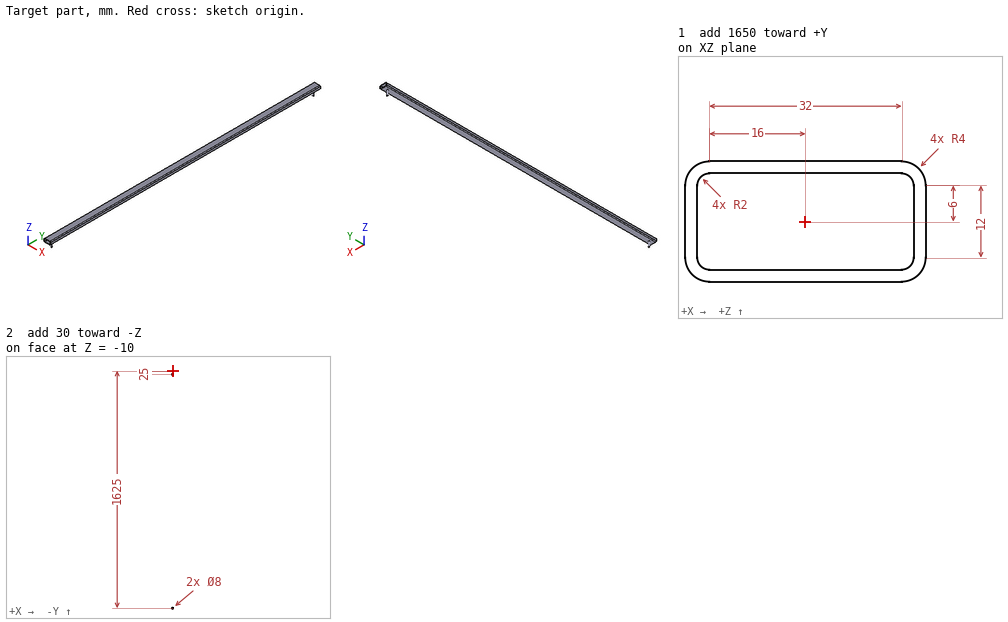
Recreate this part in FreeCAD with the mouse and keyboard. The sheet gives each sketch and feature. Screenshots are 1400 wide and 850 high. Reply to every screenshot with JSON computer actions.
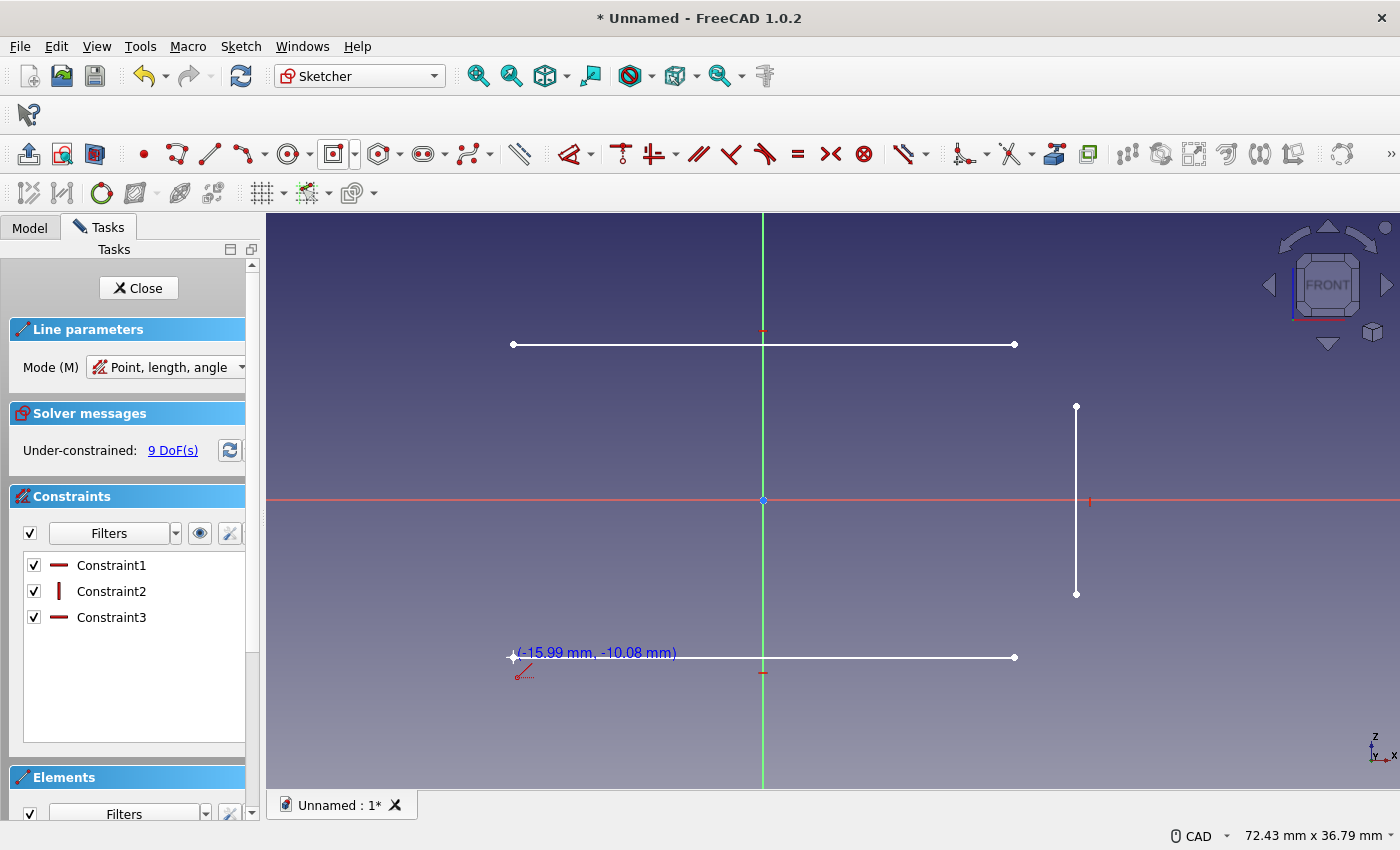
{"action": "left_click", "coordinate": [450, 594]}
{"action": "left_click", "coordinate": [450, 406]}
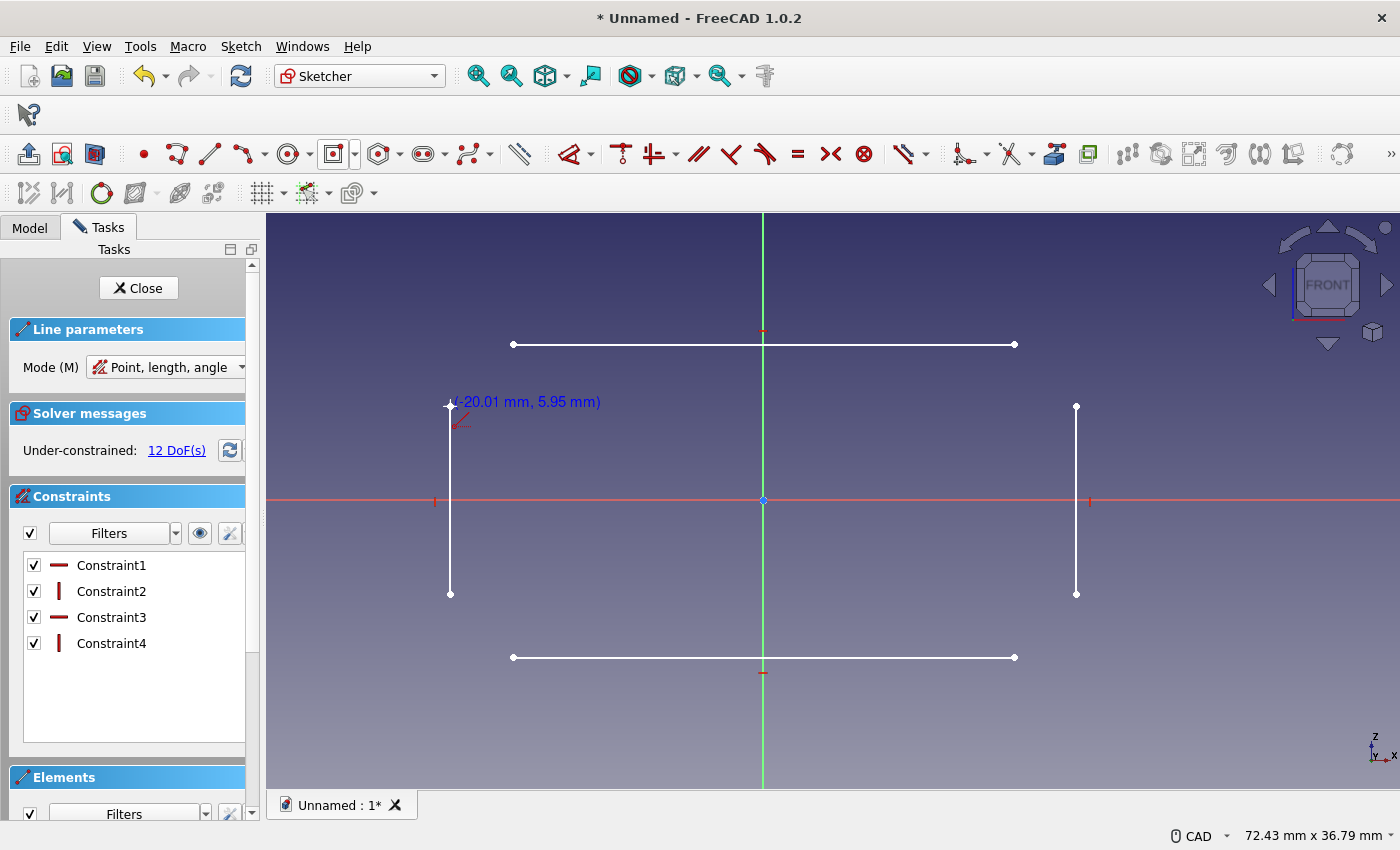
{"action": "left_click", "coordinate": [242, 154]}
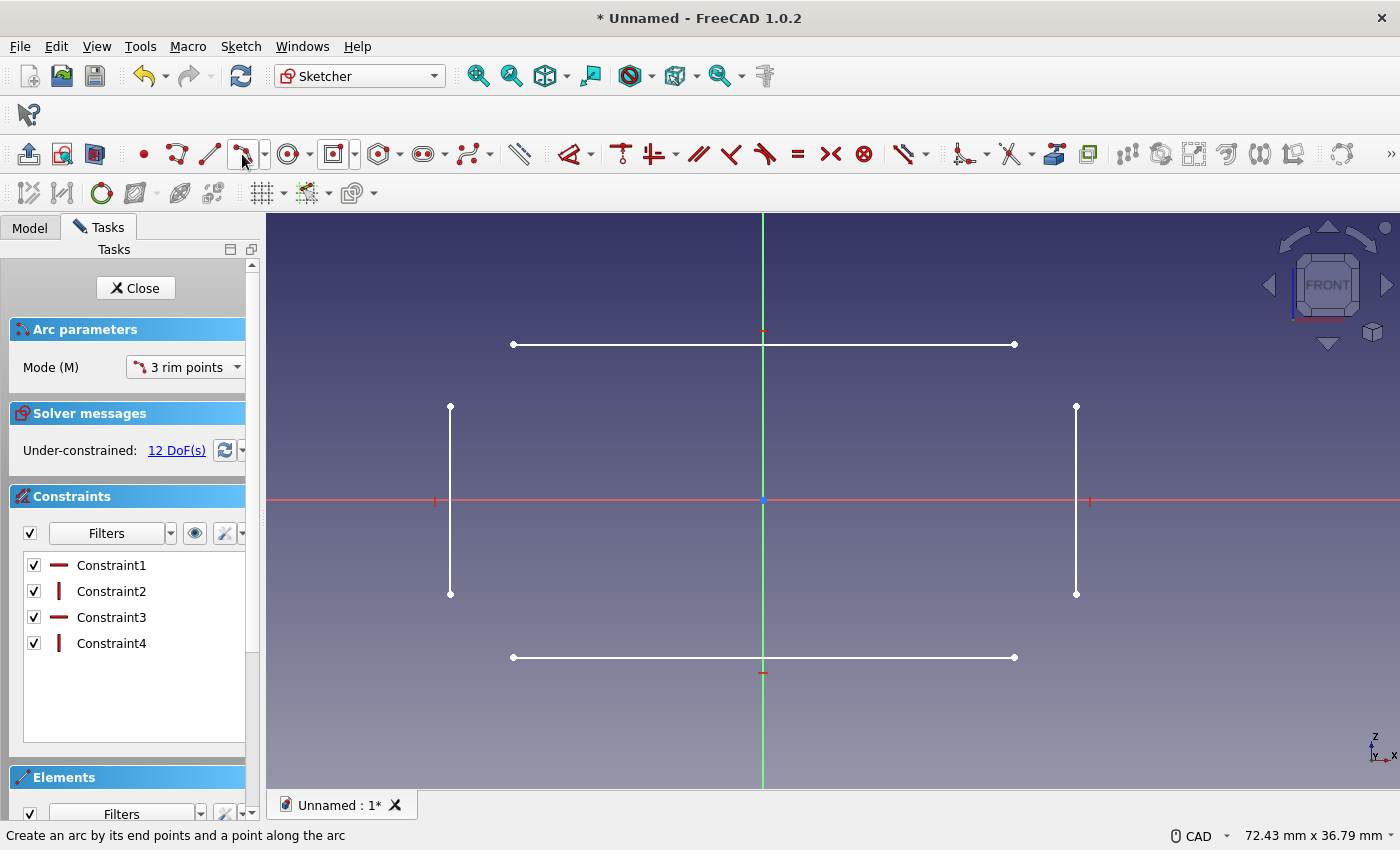
{"action": "left_click", "coordinate": [1014, 345]}
{"action": "left_click", "coordinate": [1076, 407]}
{"action": "left_click", "coordinate": [1058, 362]}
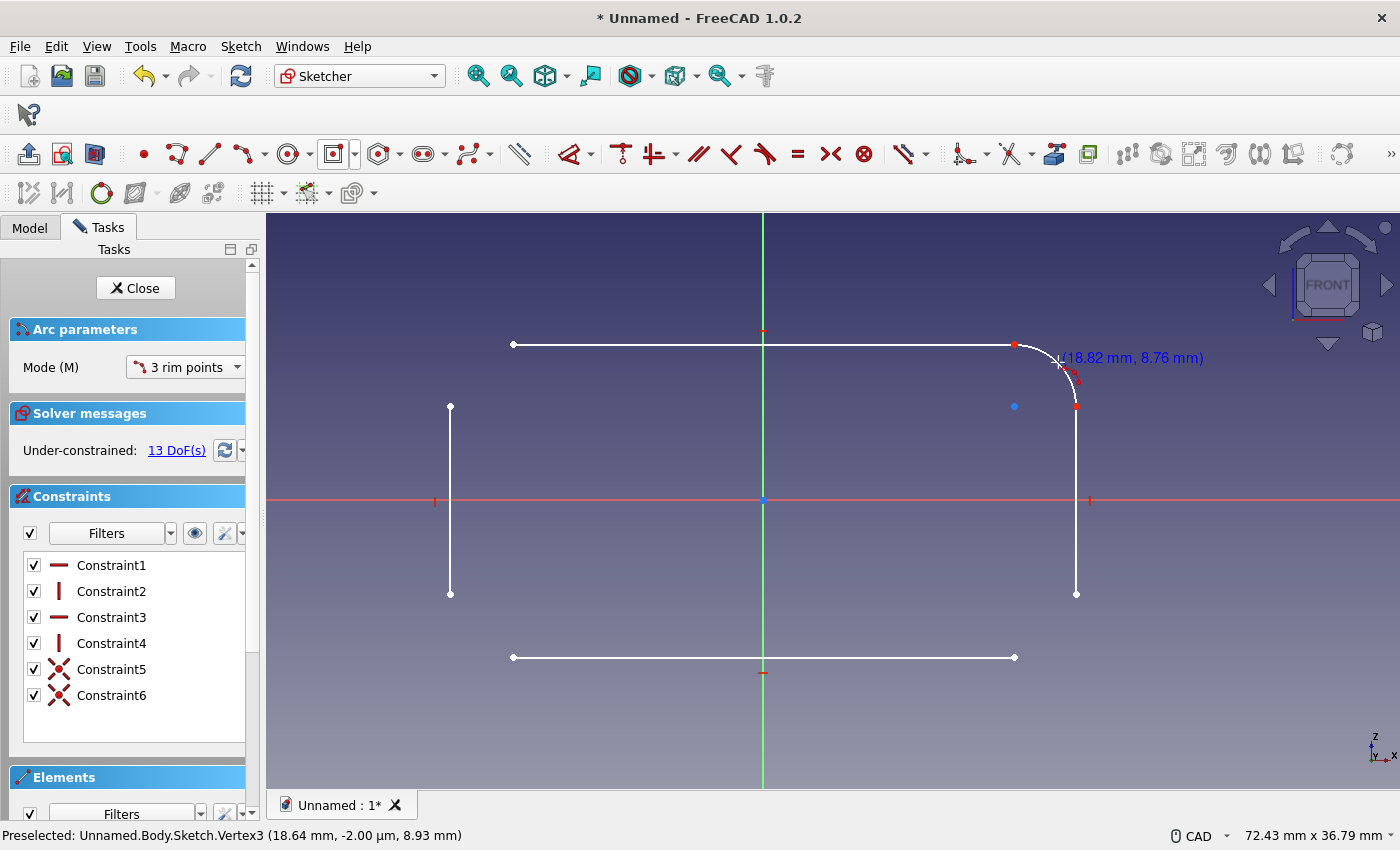
{"action": "left_click", "coordinate": [1076, 595]}
{"action": "left_click", "coordinate": [1014, 658]}
{"action": "left_click", "coordinate": [1058, 638]}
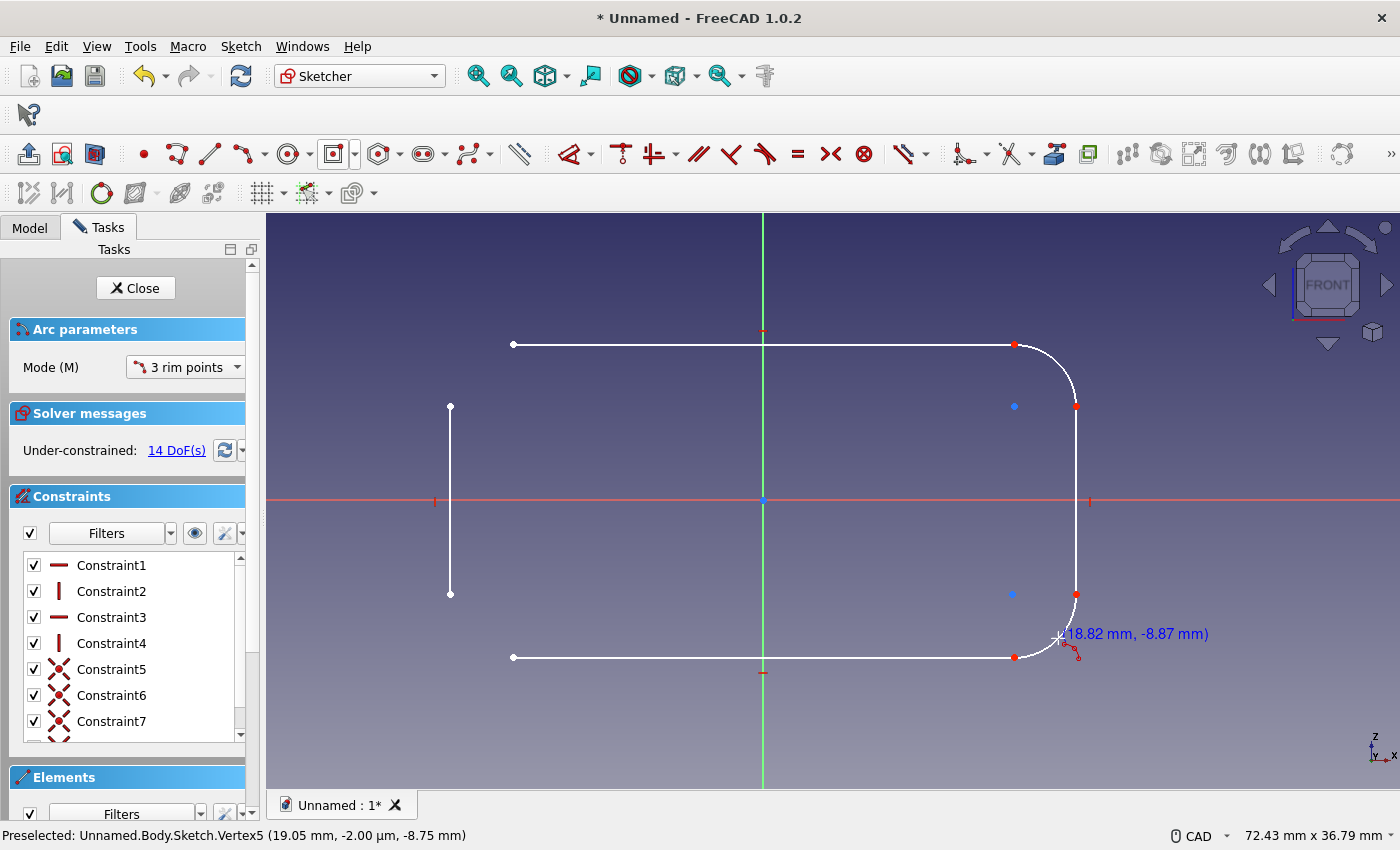
{"action": "left_click", "coordinate": [513, 658]}
{"action": "left_click", "coordinate": [450, 595]}
{"action": "left_click", "coordinate": [469, 638]}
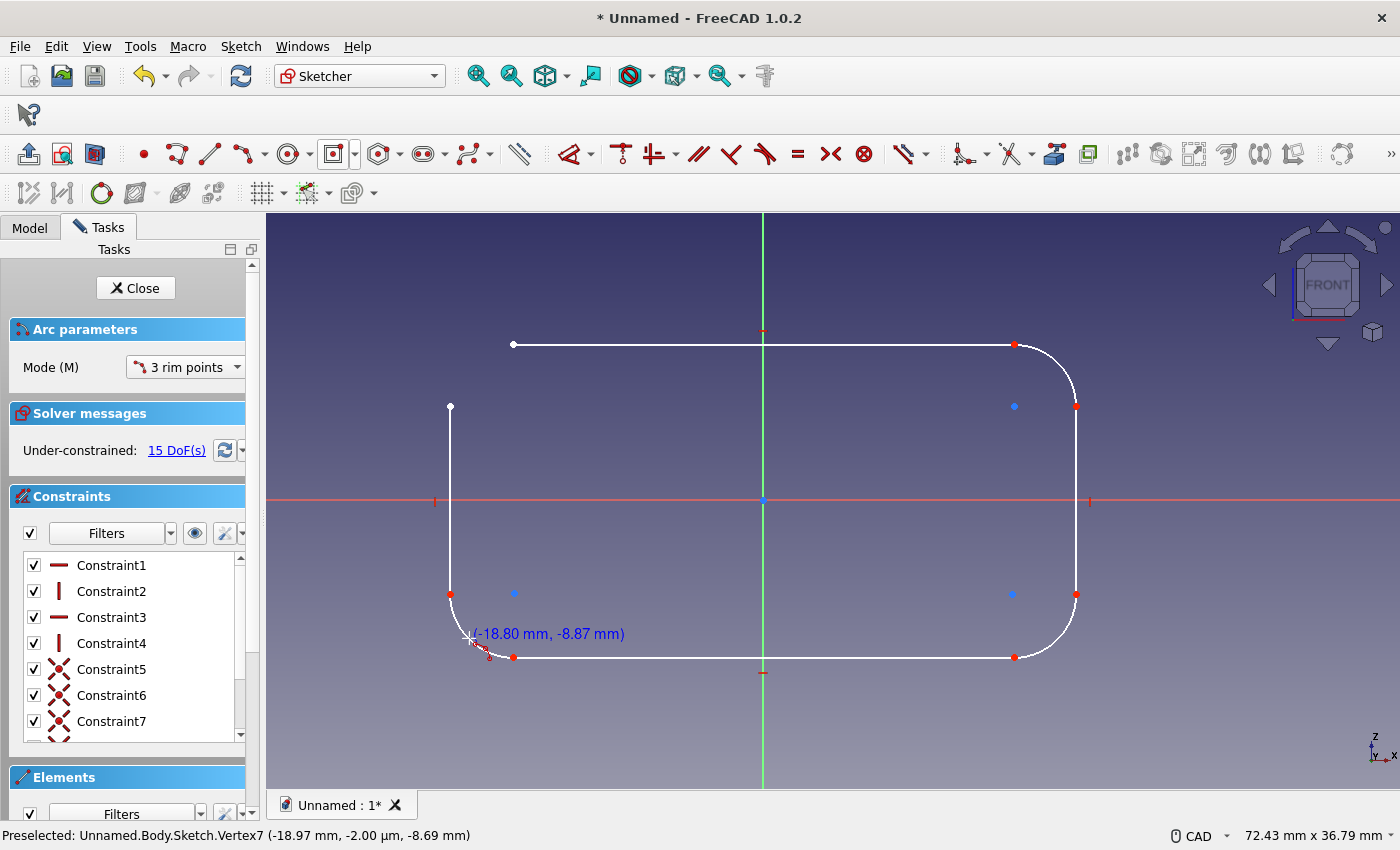
{"action": "left_click", "coordinate": [450, 407]}
{"action": "left_click", "coordinate": [513, 345]}
{"action": "left_click", "coordinate": [469, 362]}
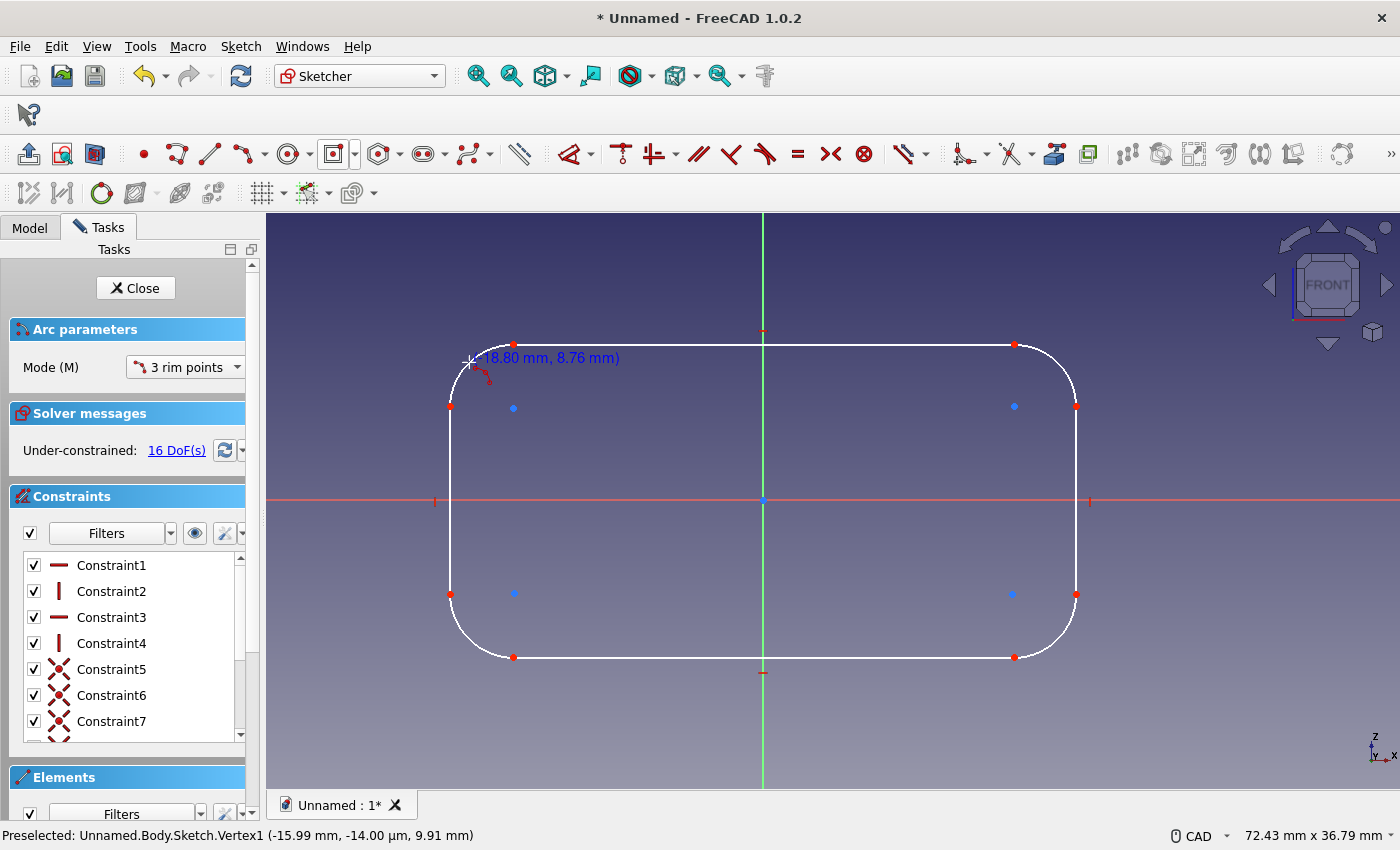
{"action": "key", "text": "g l"}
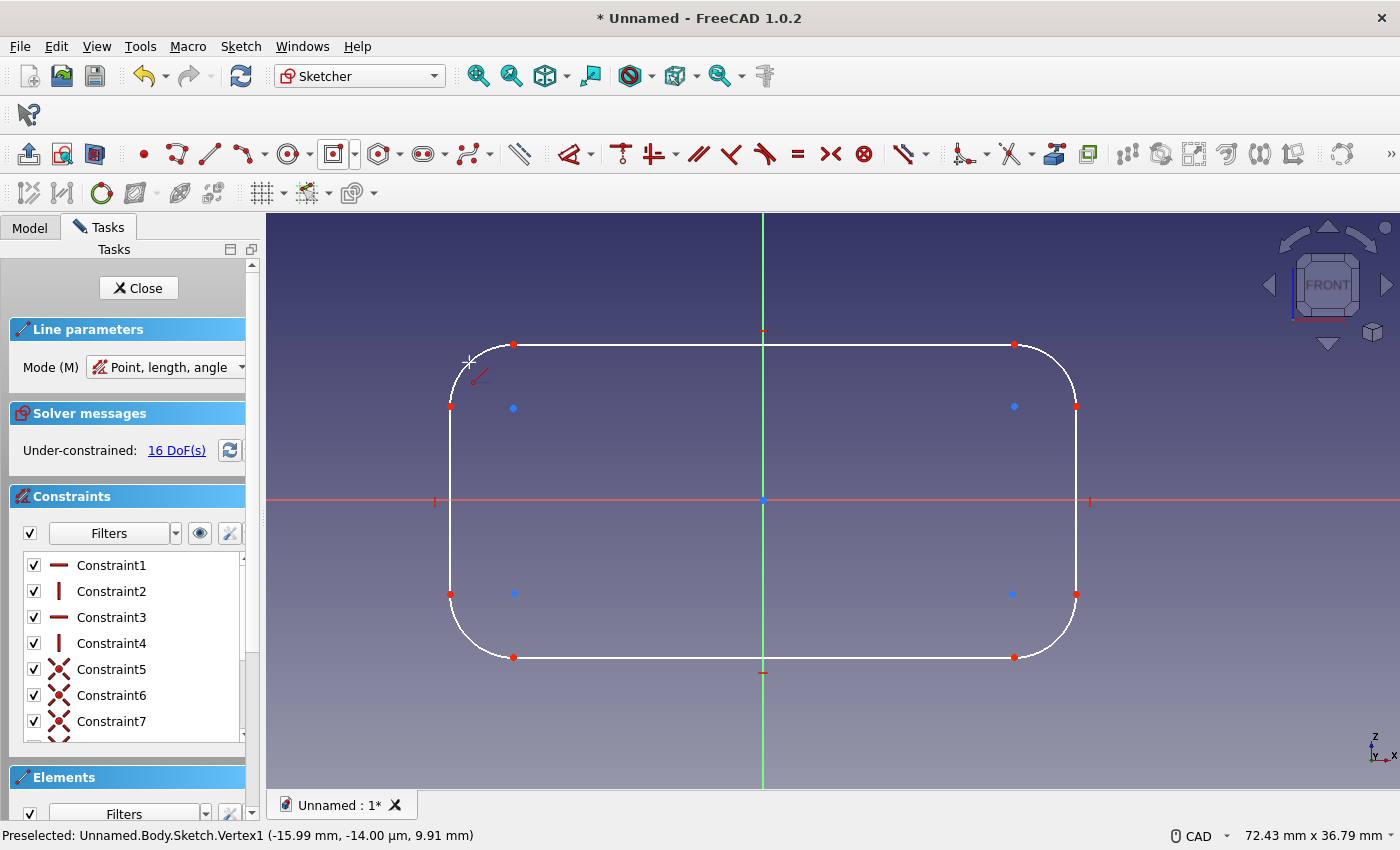
{"action": "left_click", "coordinate": [1014, 375]}
{"action": "left_click", "coordinate": [513, 375]}